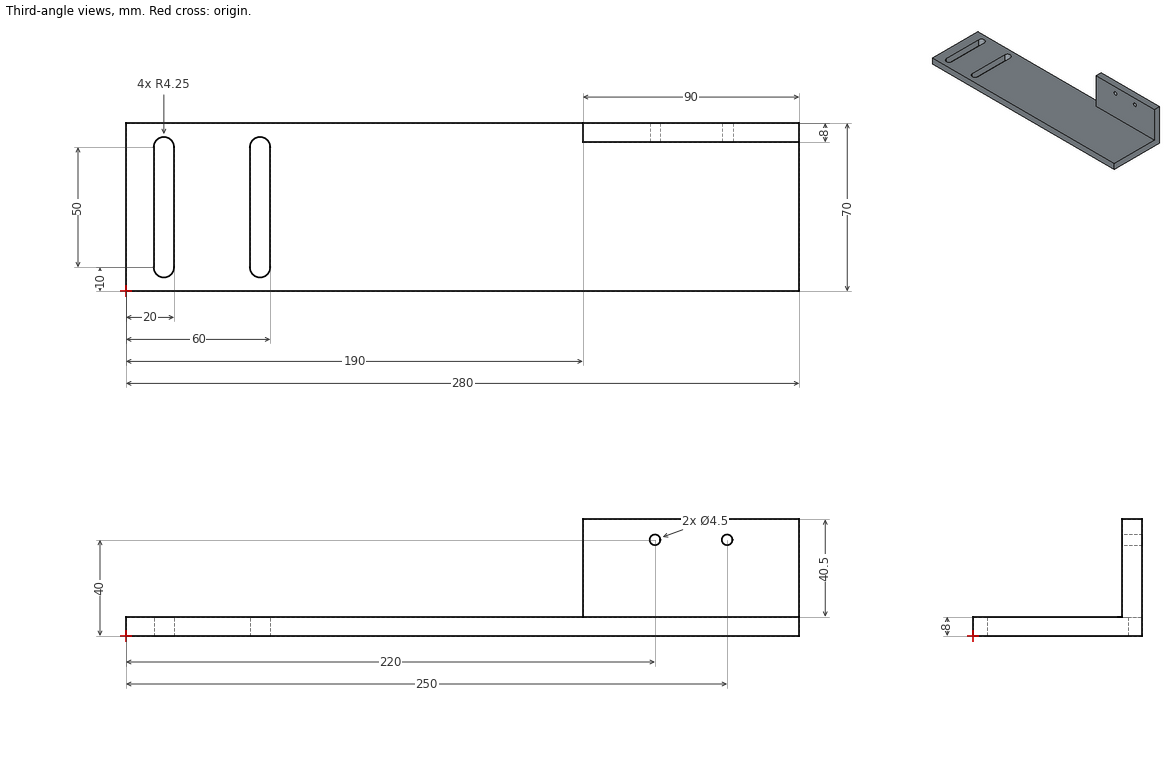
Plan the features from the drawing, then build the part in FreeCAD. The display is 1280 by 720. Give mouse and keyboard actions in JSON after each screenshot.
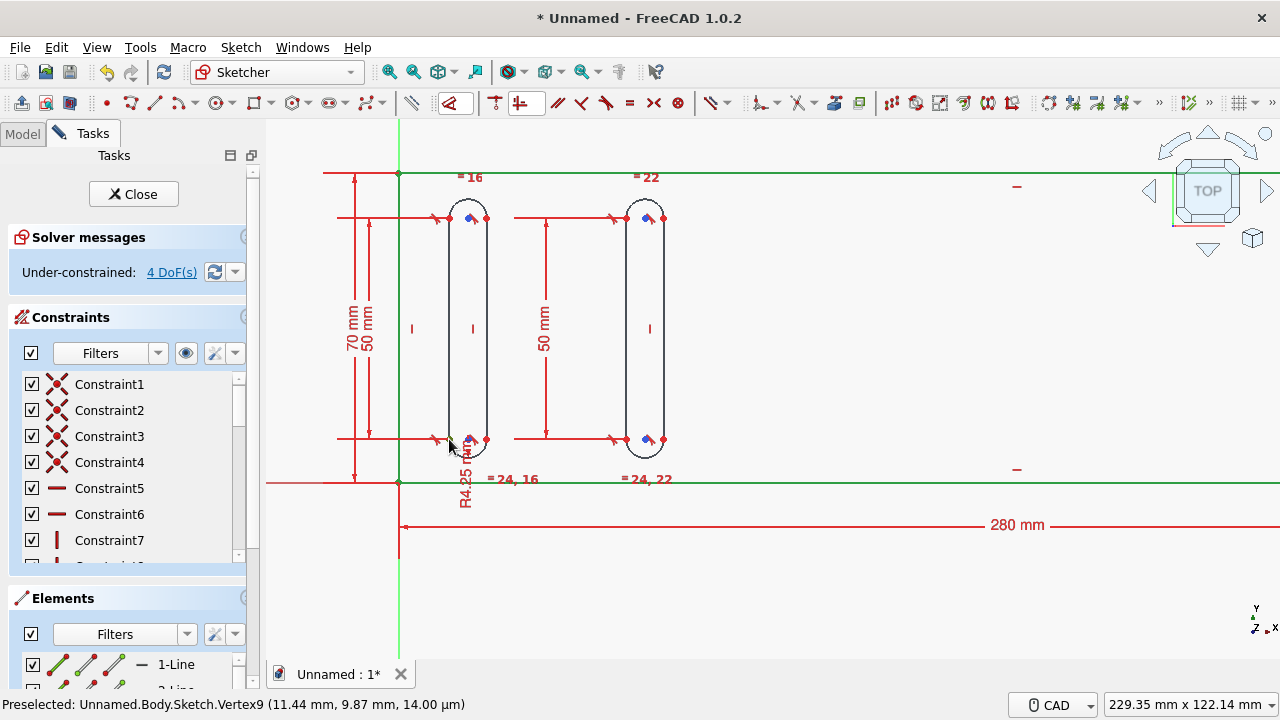
{"action": "key", "text": "i"}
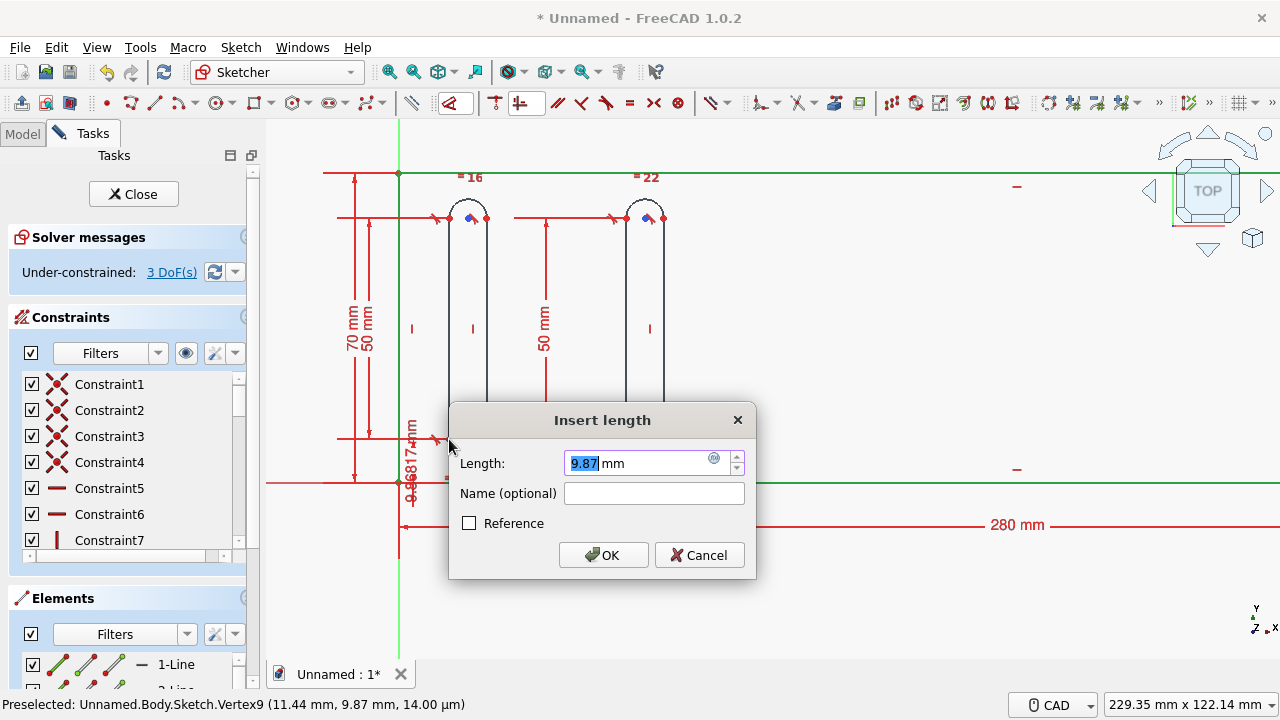
{"action": "type", "text": "10"}
{"action": "key", "text": "Return"}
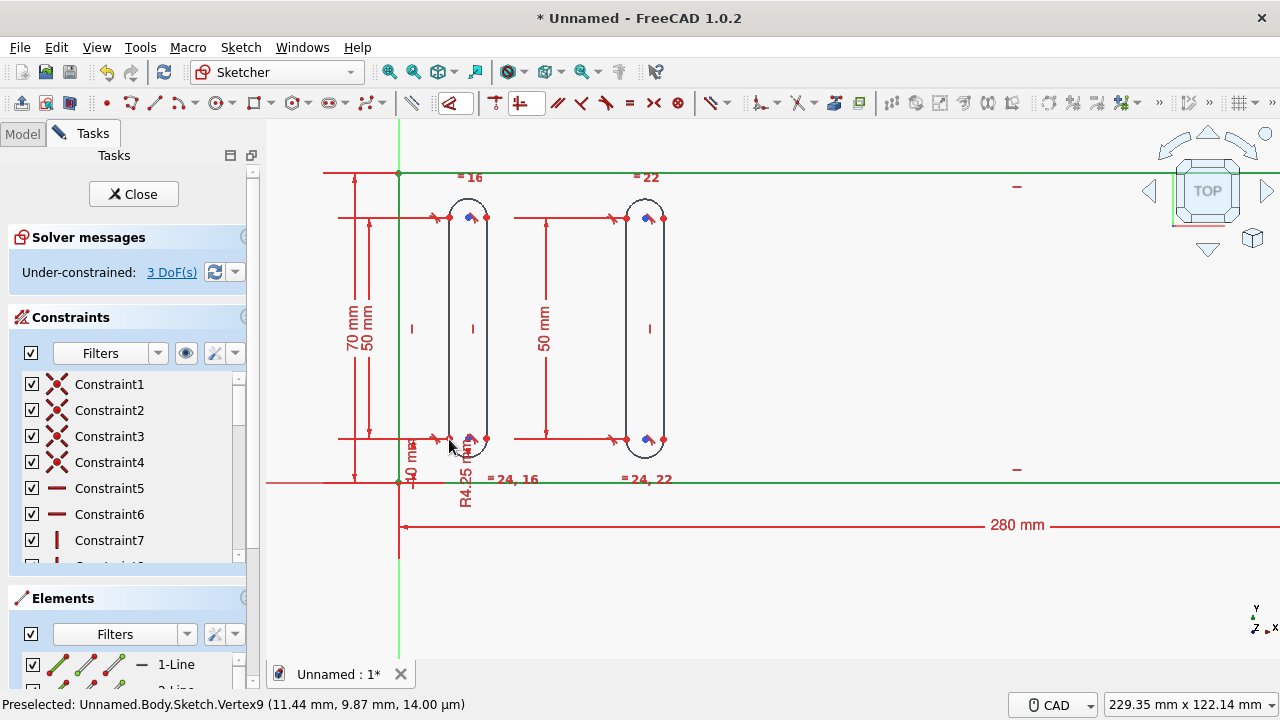
{"action": "left_click", "coordinate": [487, 439]}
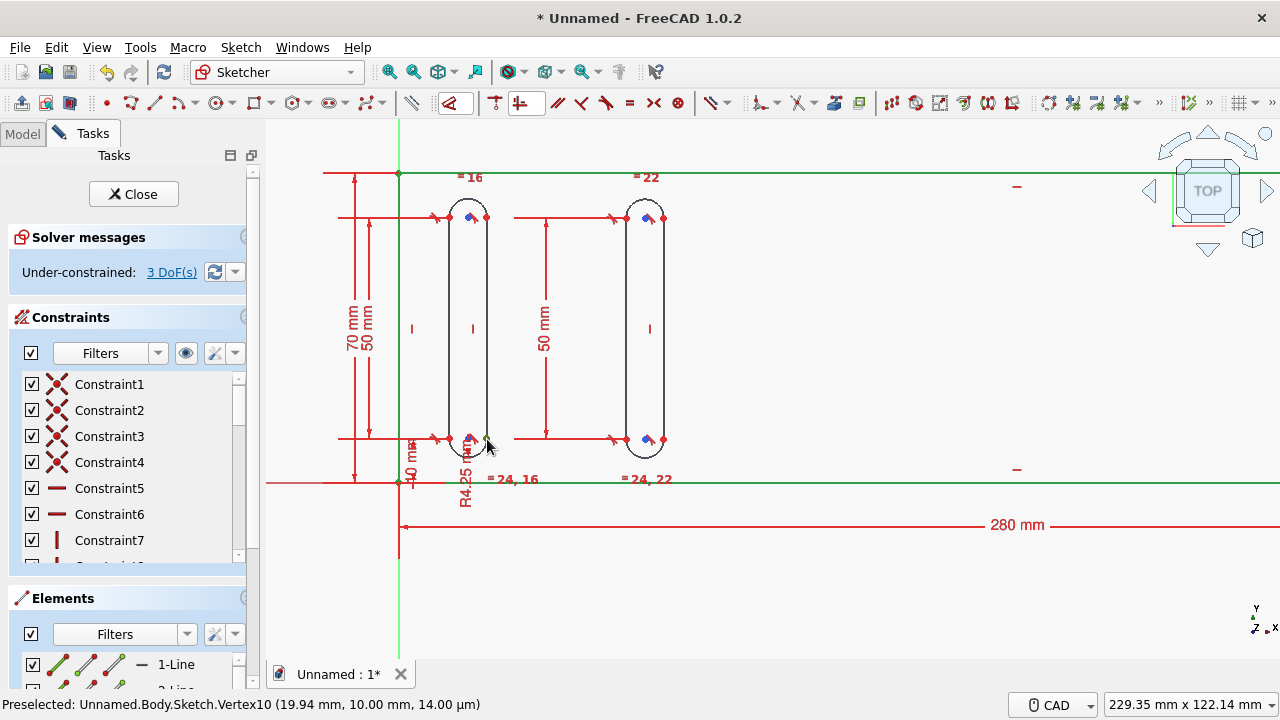
{"action": "left_click", "coordinate": [468, 104]}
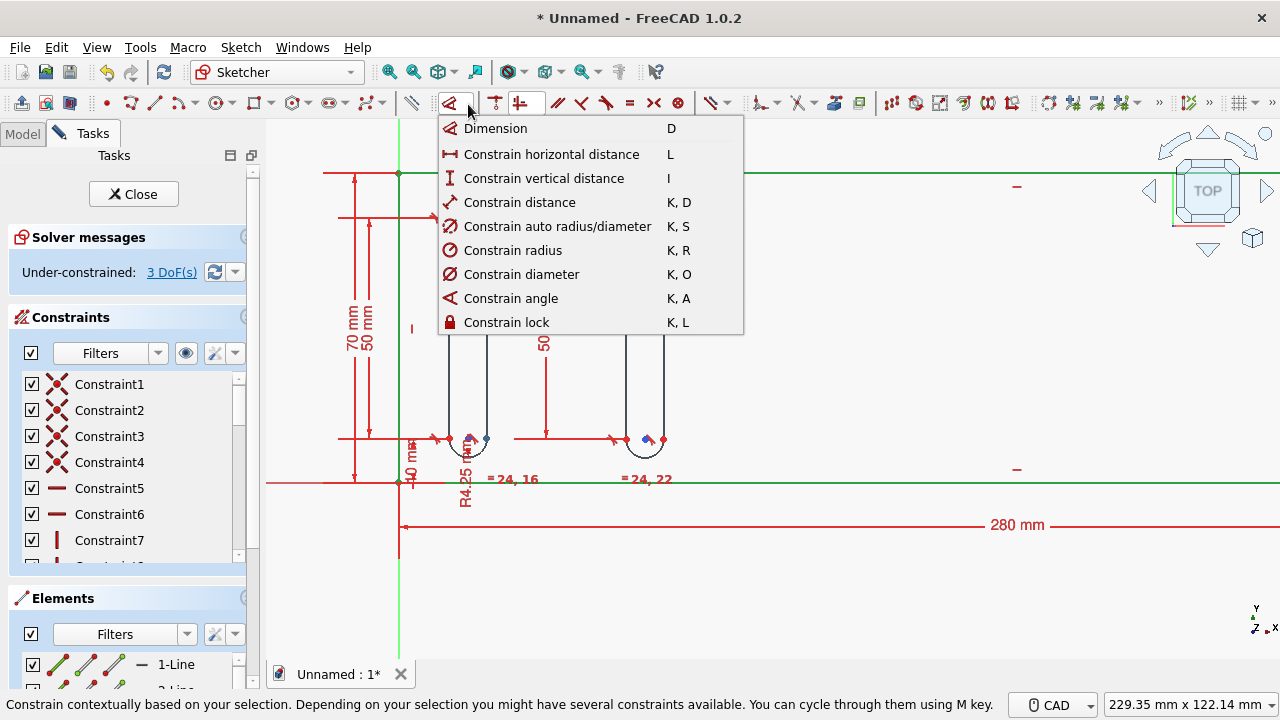
{"action": "left_click", "coordinate": [591, 154]}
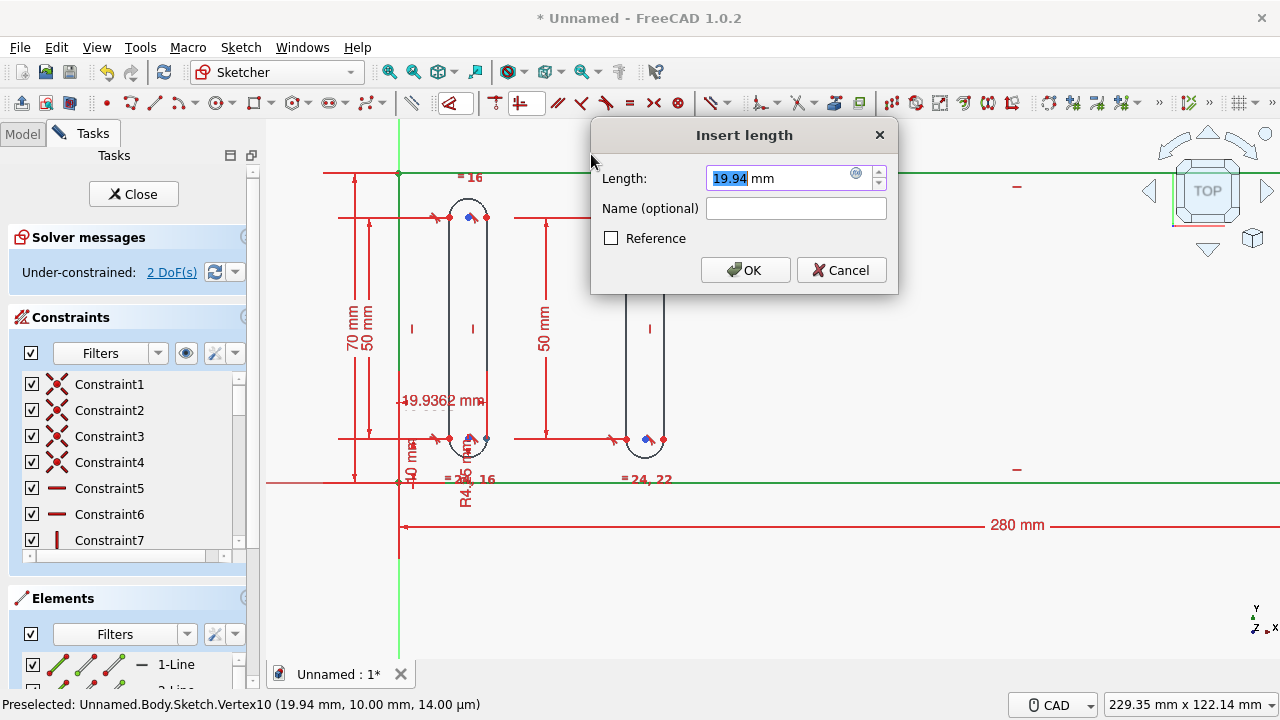
{"action": "type", "text": "20"}
{"action": "key", "text": "Return"}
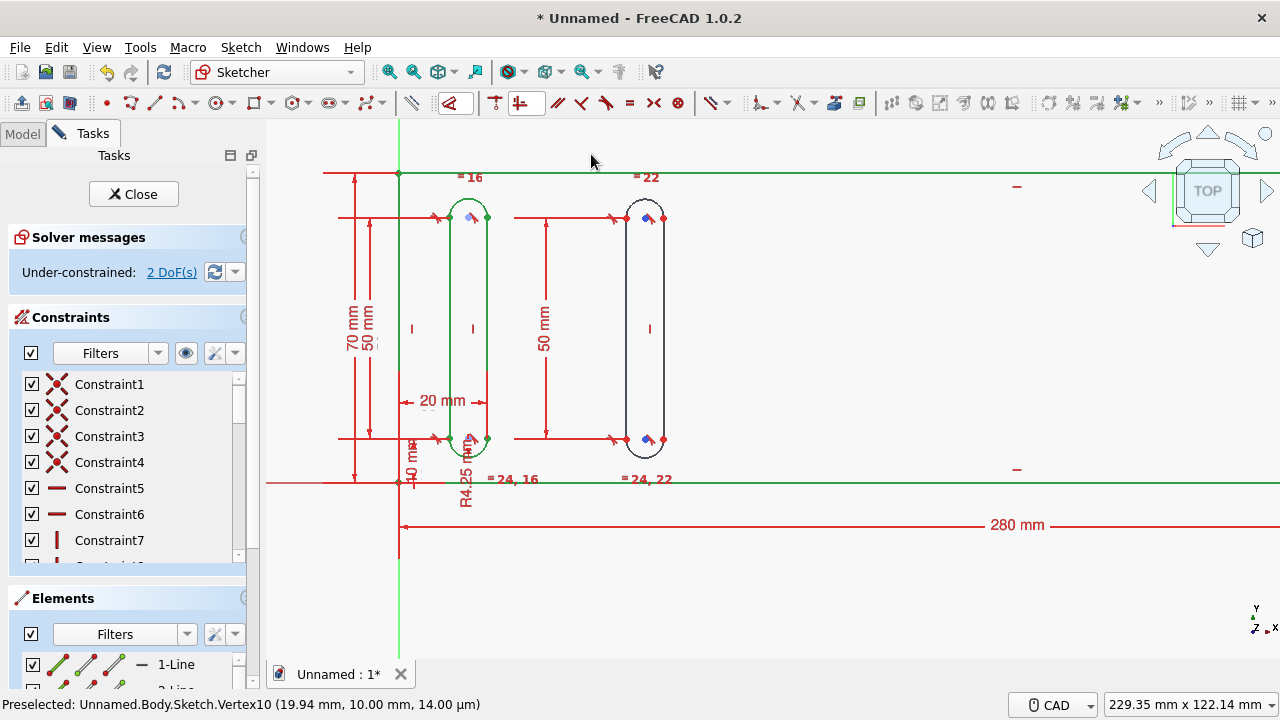
{"action": "left_click", "coordinate": [626, 439]}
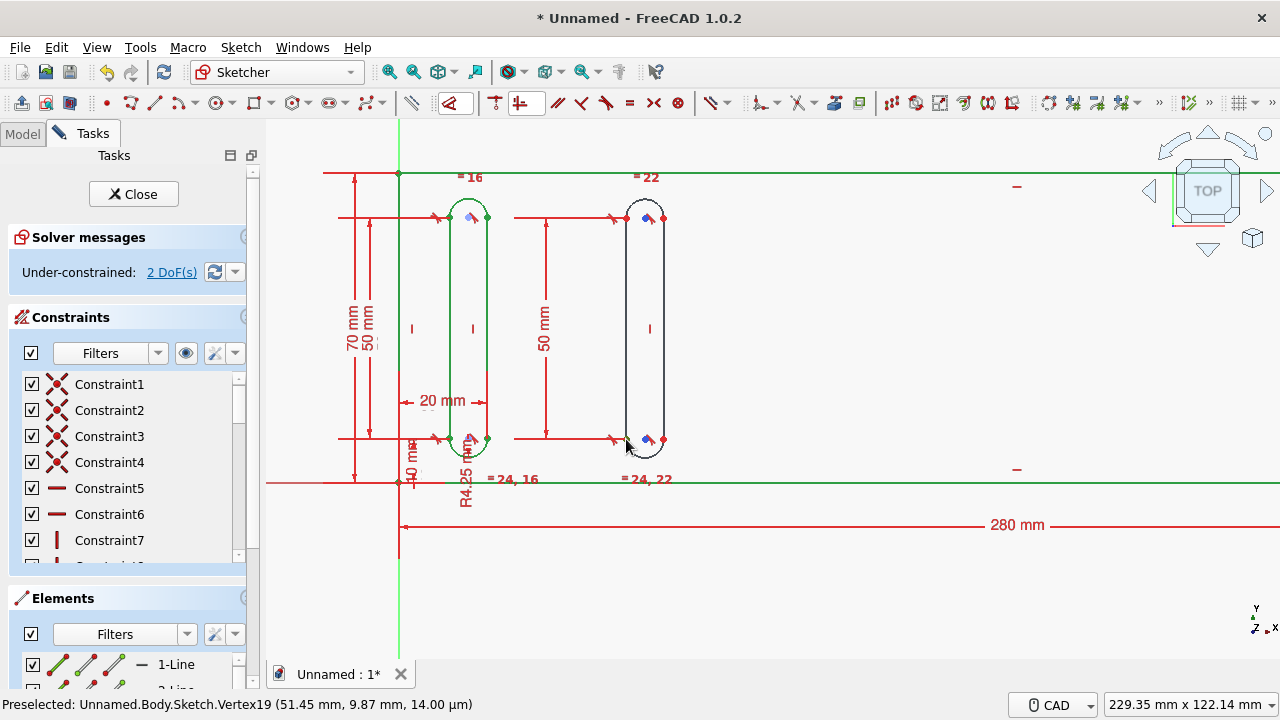
{"action": "key", "text": "i"}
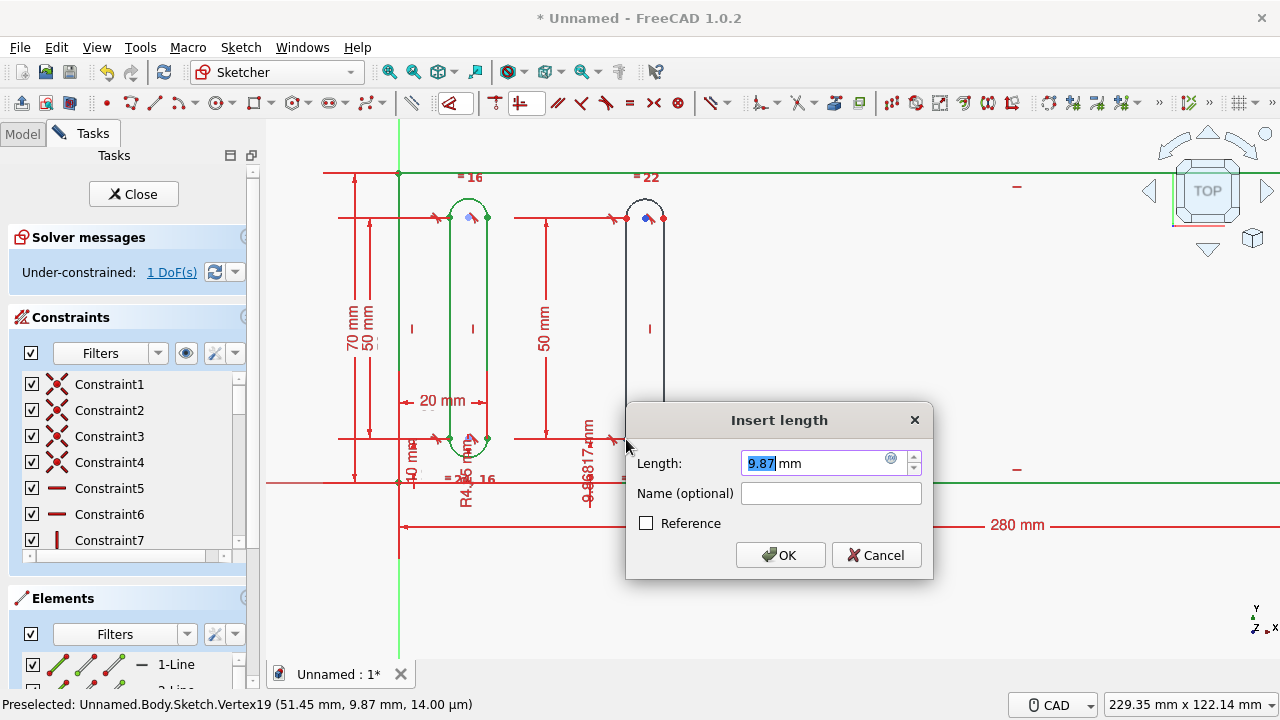
{"action": "type", "text": "10"}
{"action": "key", "text": "Return"}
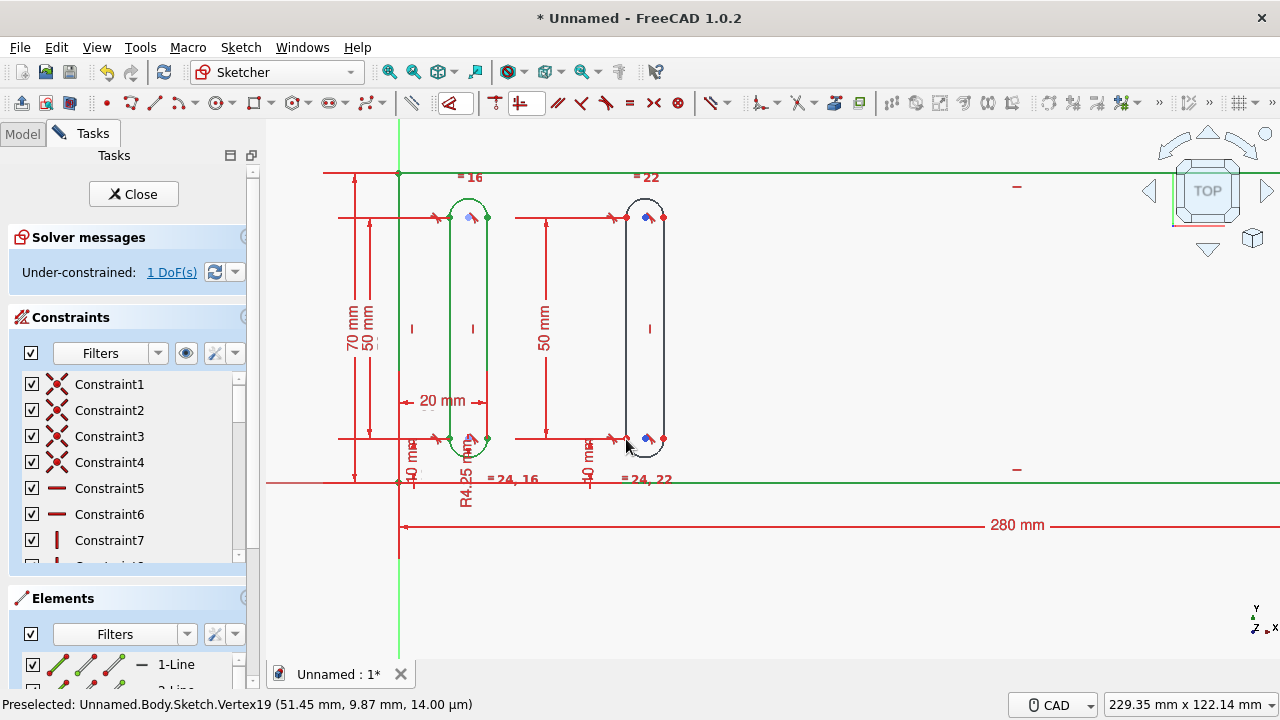
{"action": "left_click", "coordinate": [664, 439]}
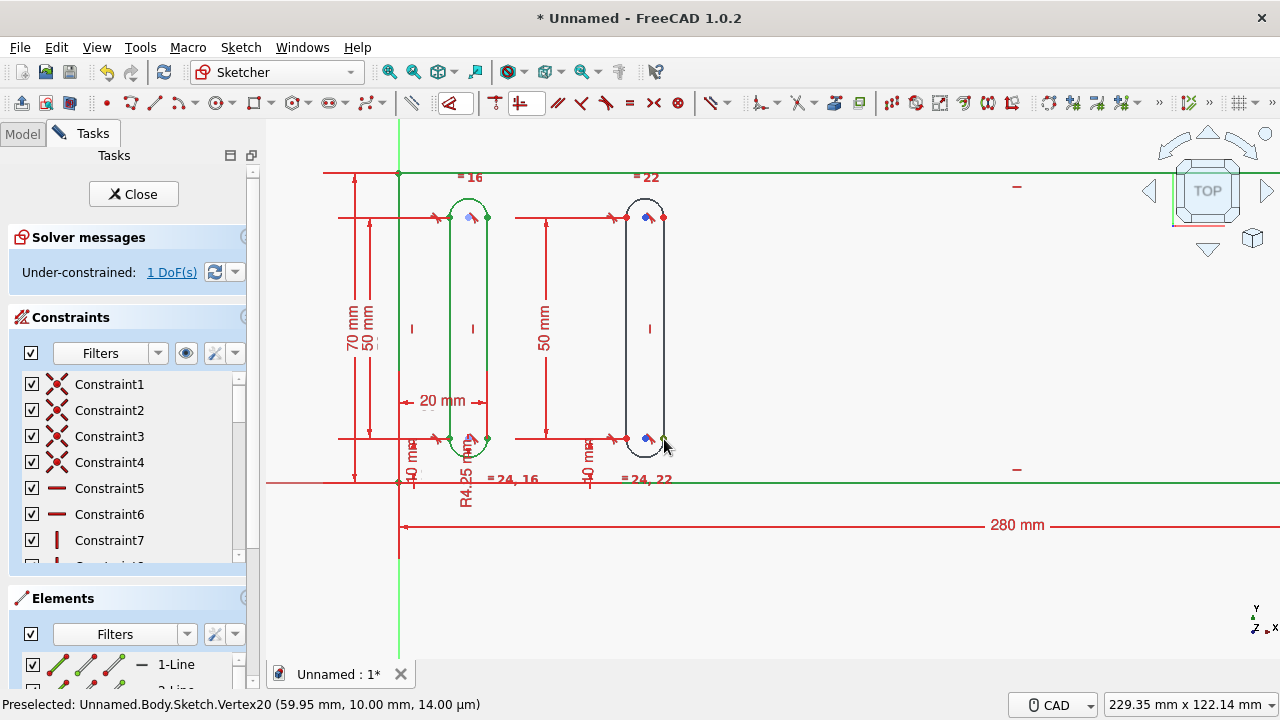
{"action": "key", "text": "l"}